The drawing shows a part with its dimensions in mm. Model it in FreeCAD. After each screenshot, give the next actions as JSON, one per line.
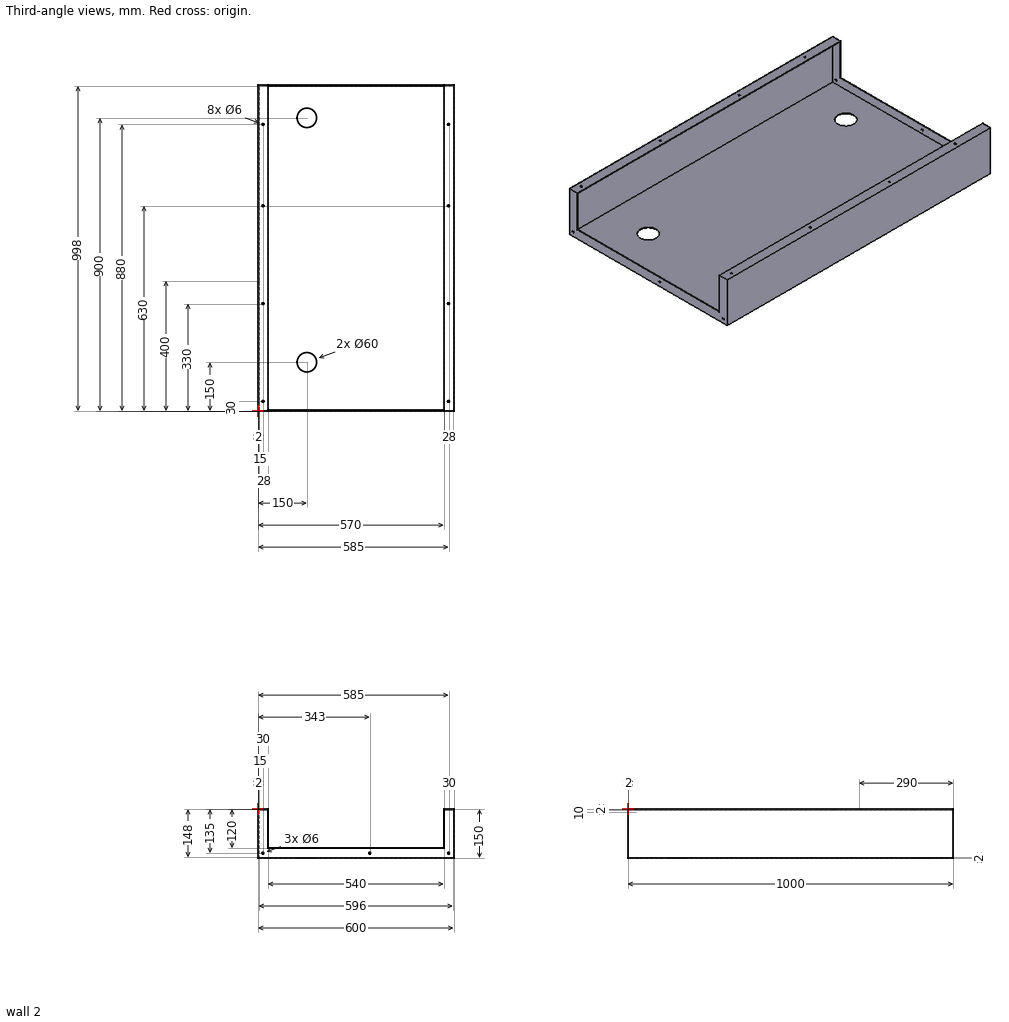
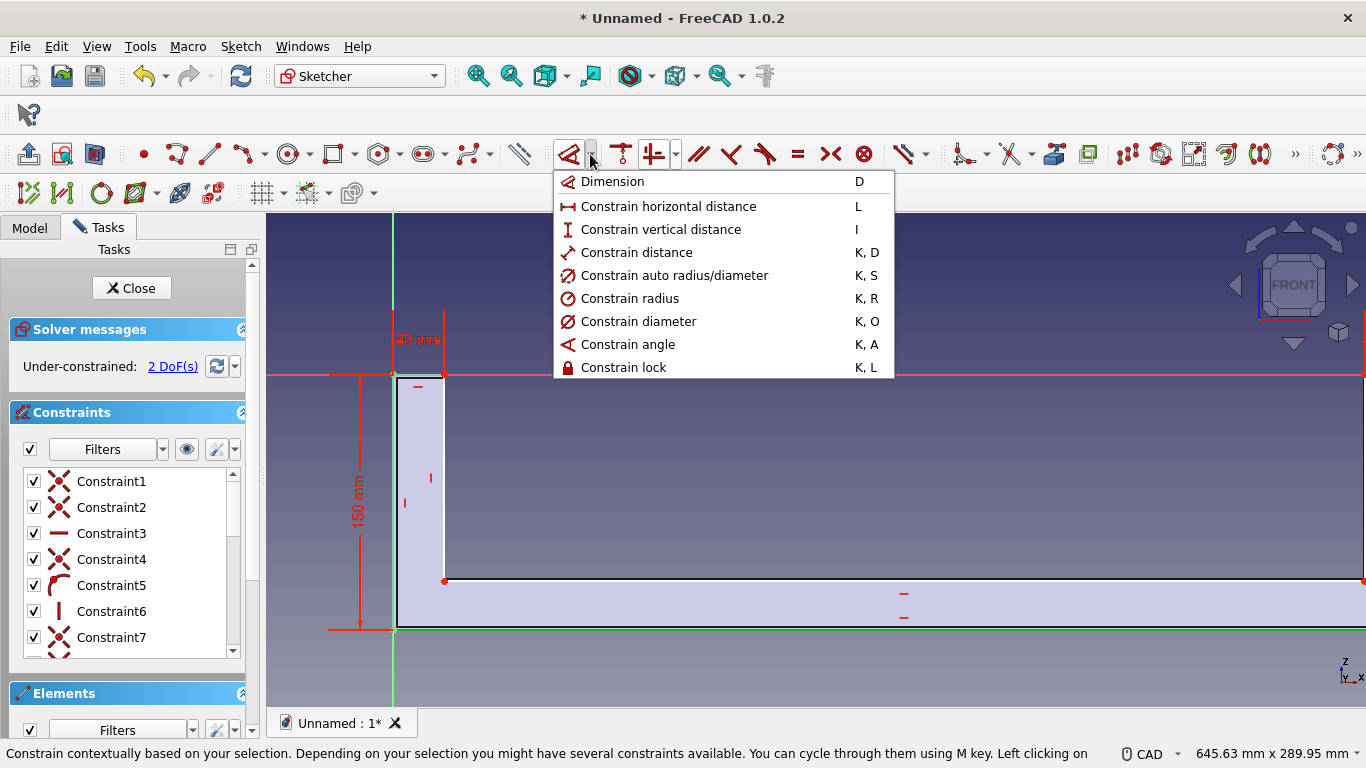
{"action": "left_click", "coordinate": [724, 206]}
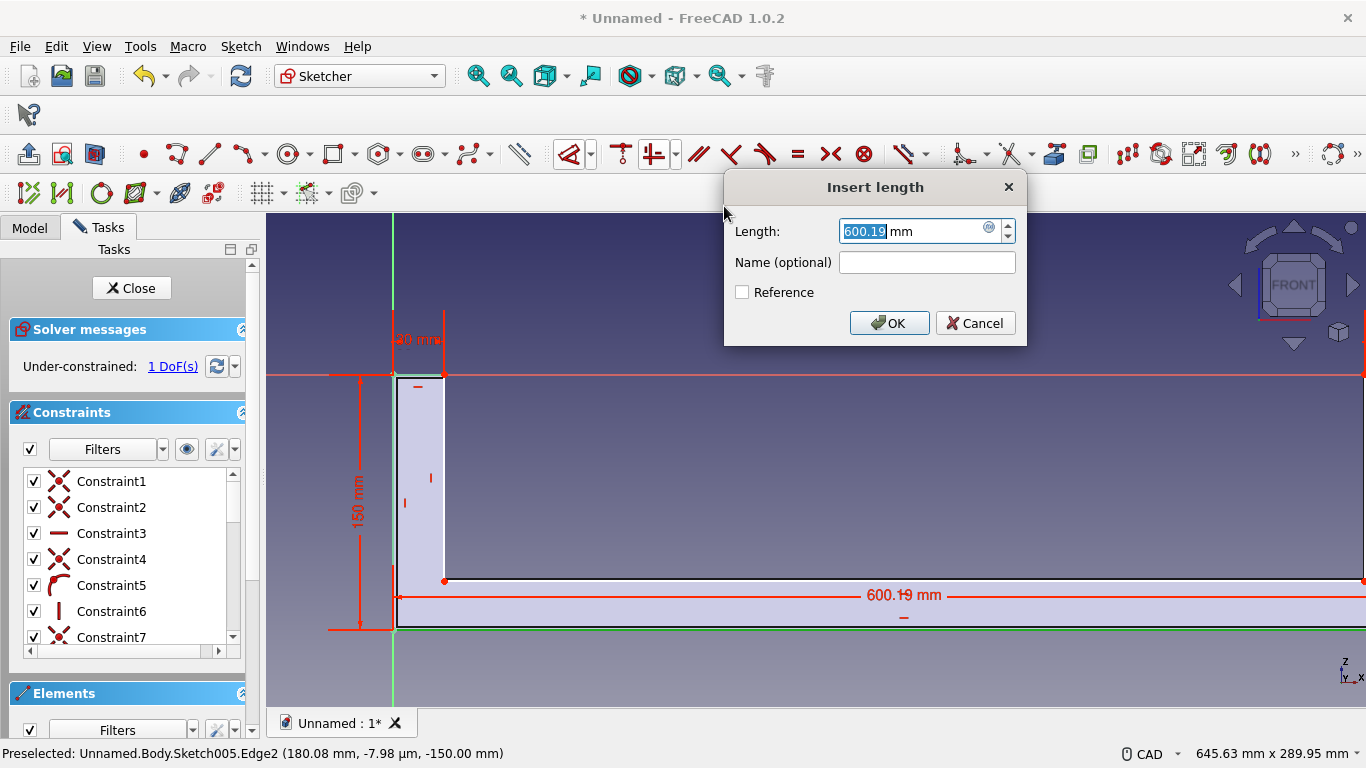
{"action": "type", "text": "600"}
{"action": "key", "text": "Return"}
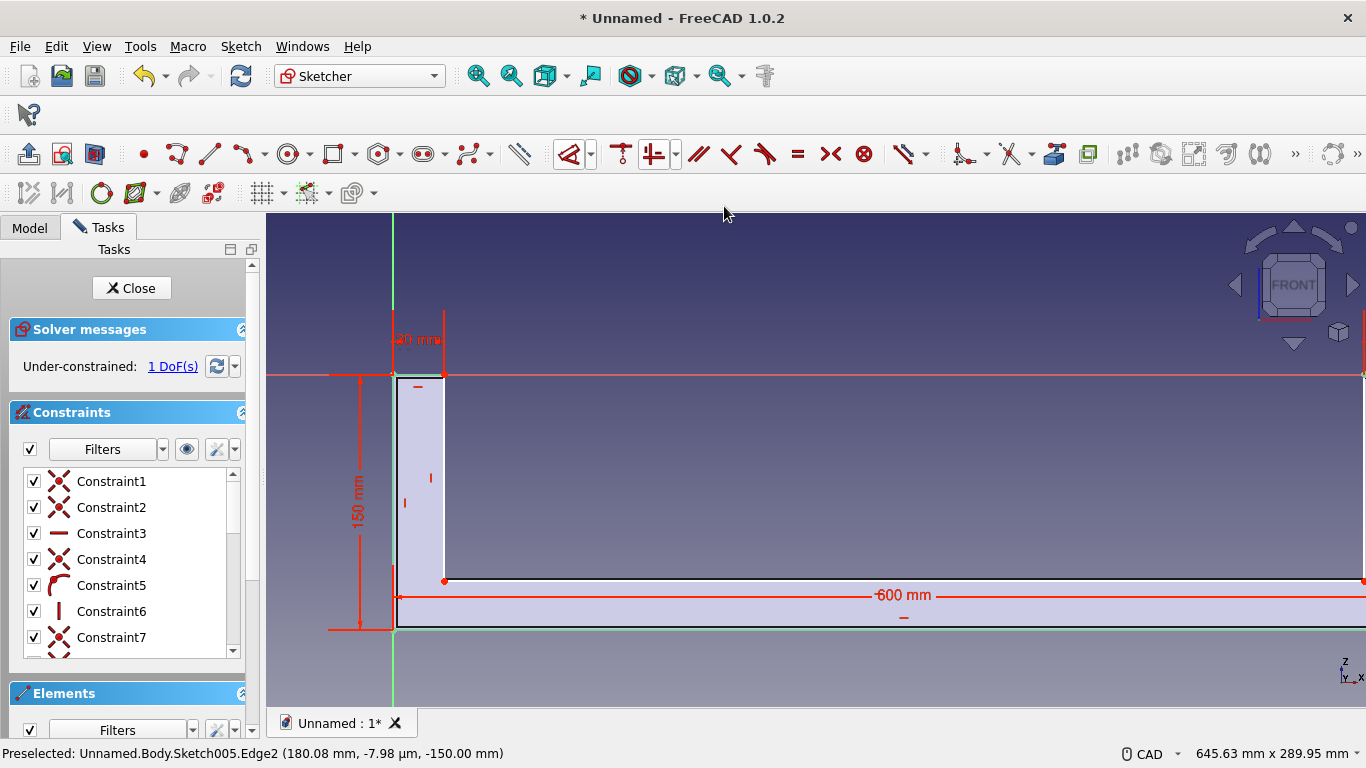
{"action": "scroll", "coordinate": [429, 374], "scroll_direction": "down", "scroll_amount": 2}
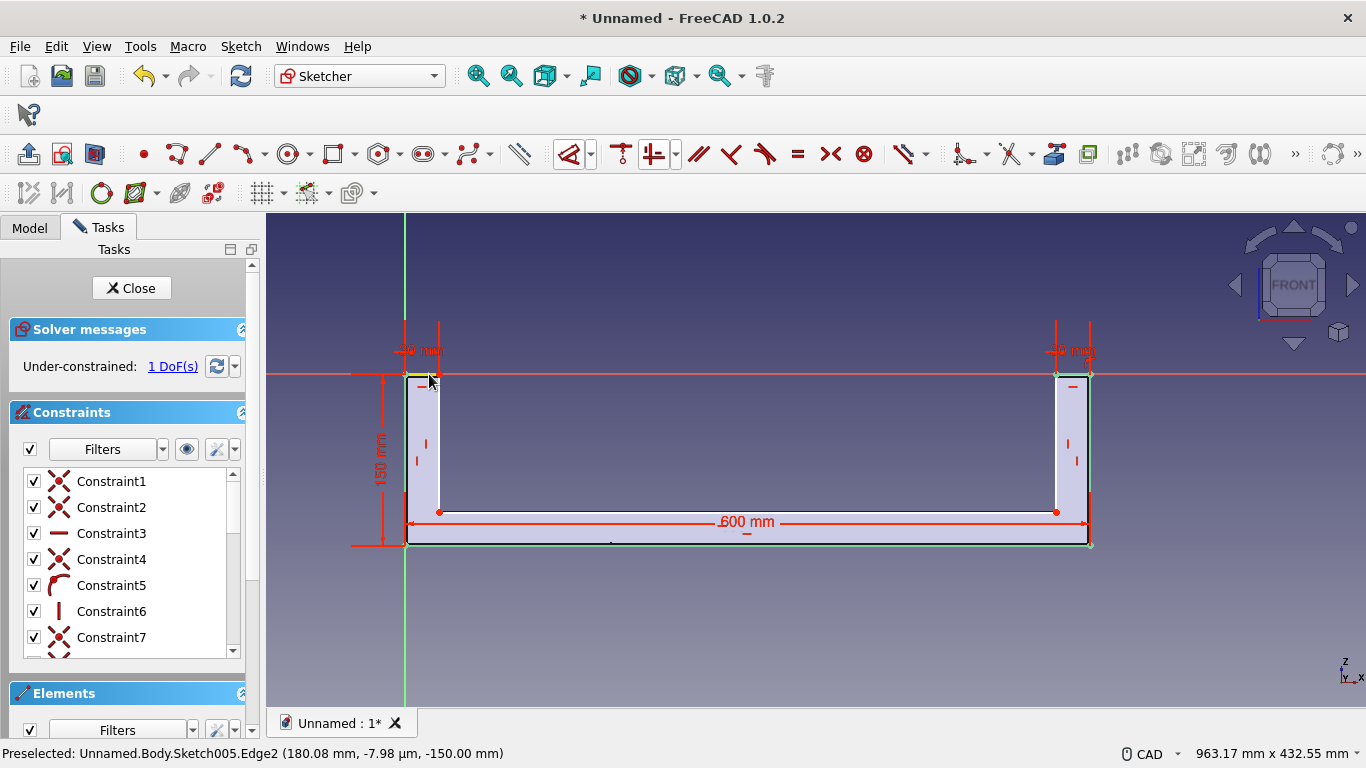
{"action": "left_click", "coordinate": [1056, 416]}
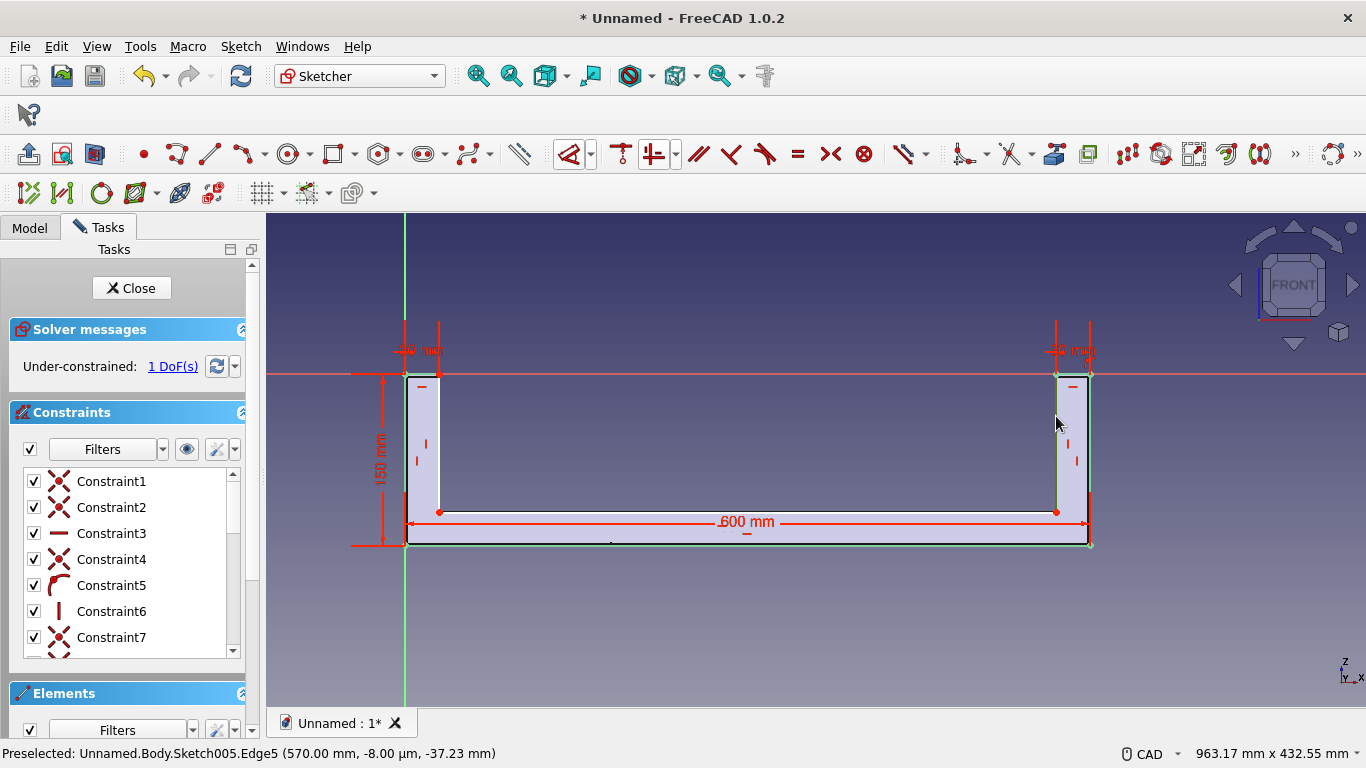
{"action": "left_click", "coordinate": [590, 154]}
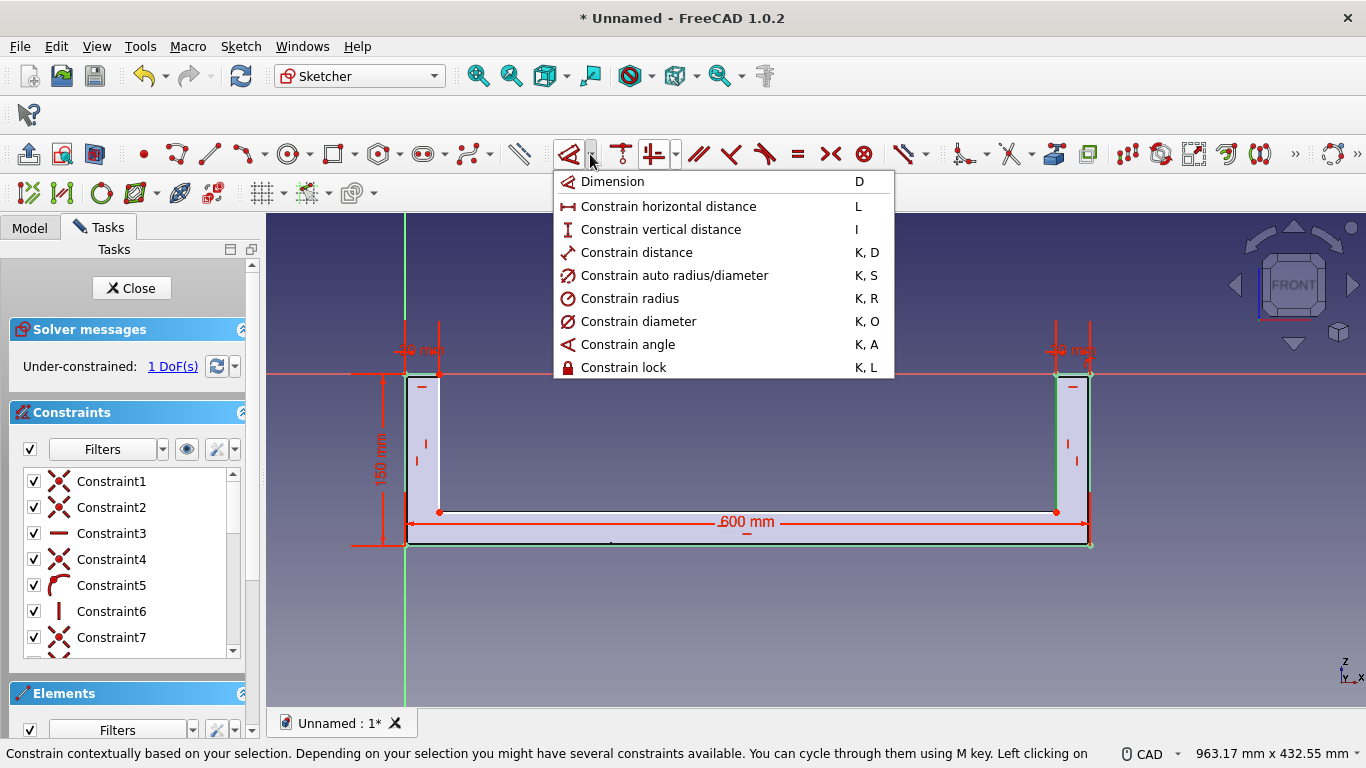
{"action": "left_click", "coordinate": [724, 230]}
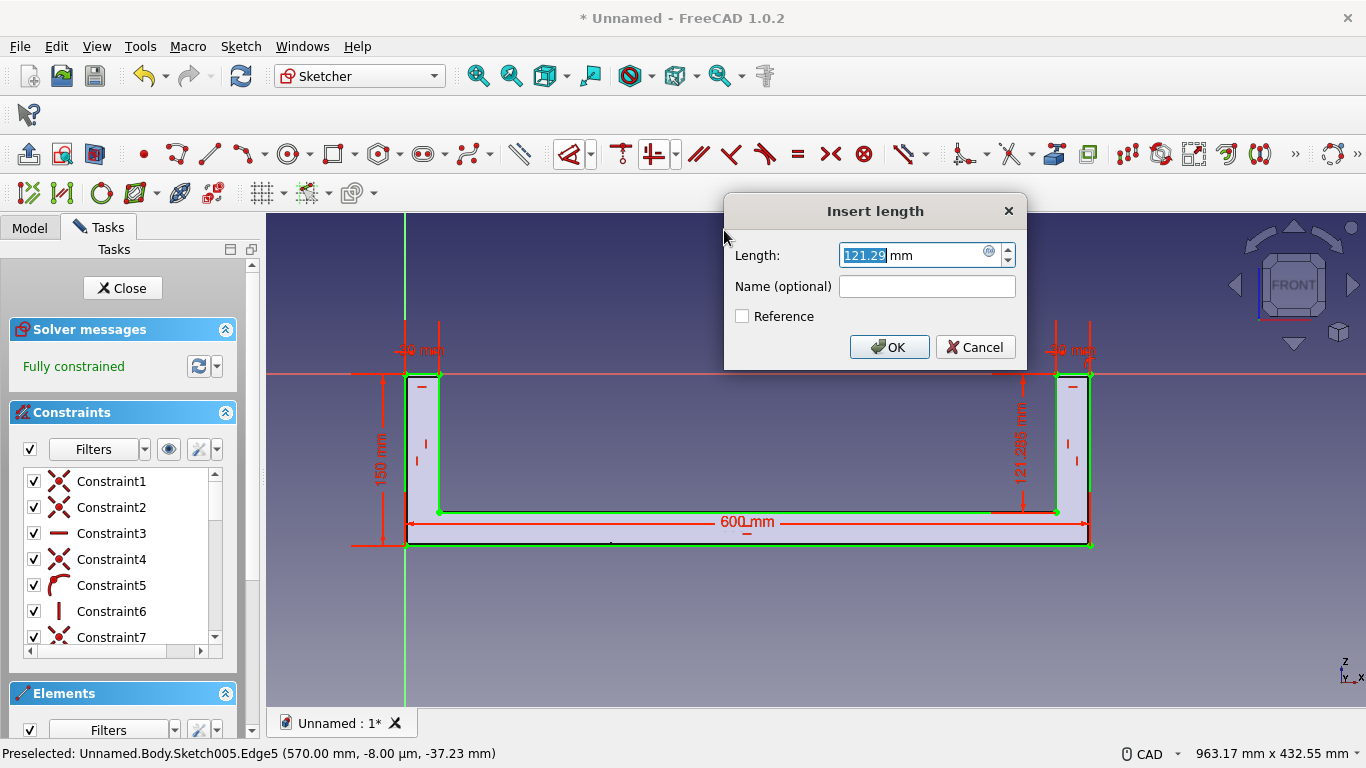
{"action": "type", "text": "120"}
{"action": "key", "text": "Return"}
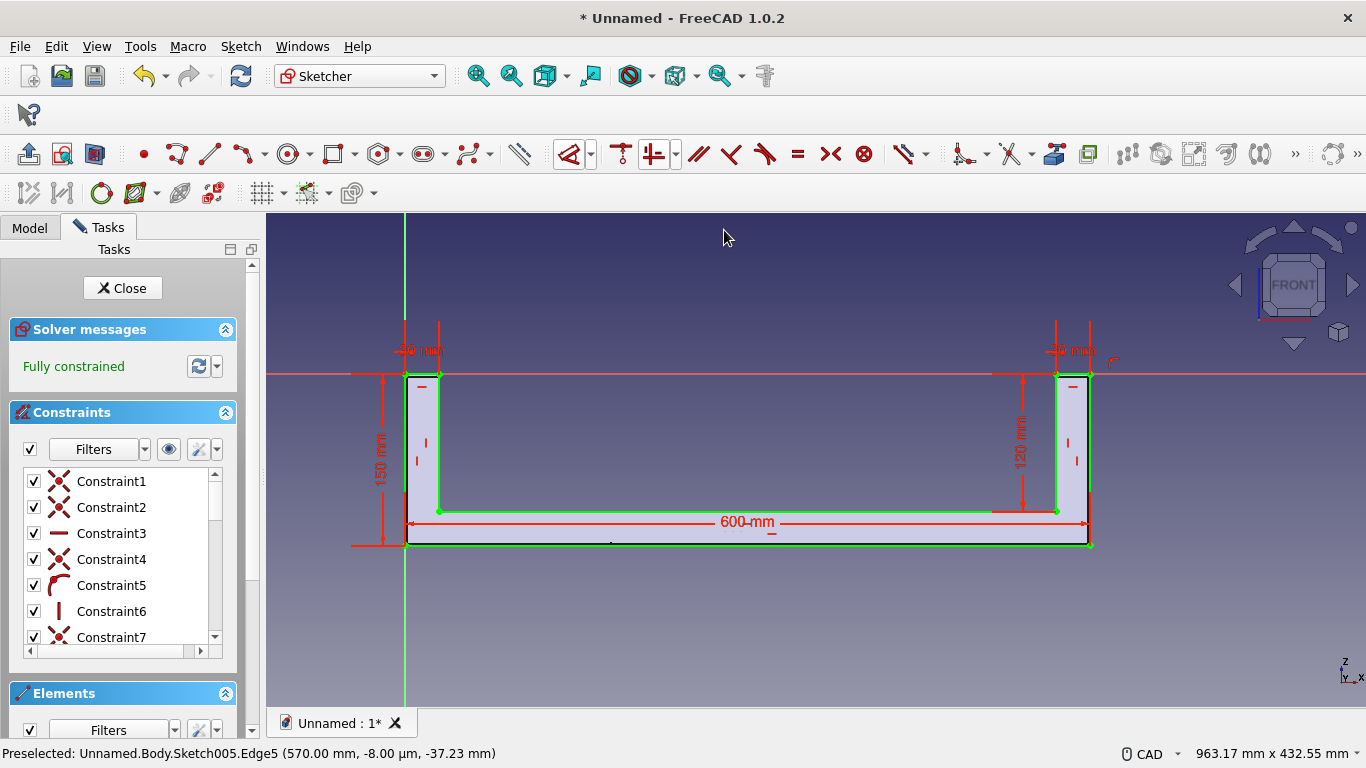
{"action": "left_click", "coordinate": [123, 288]}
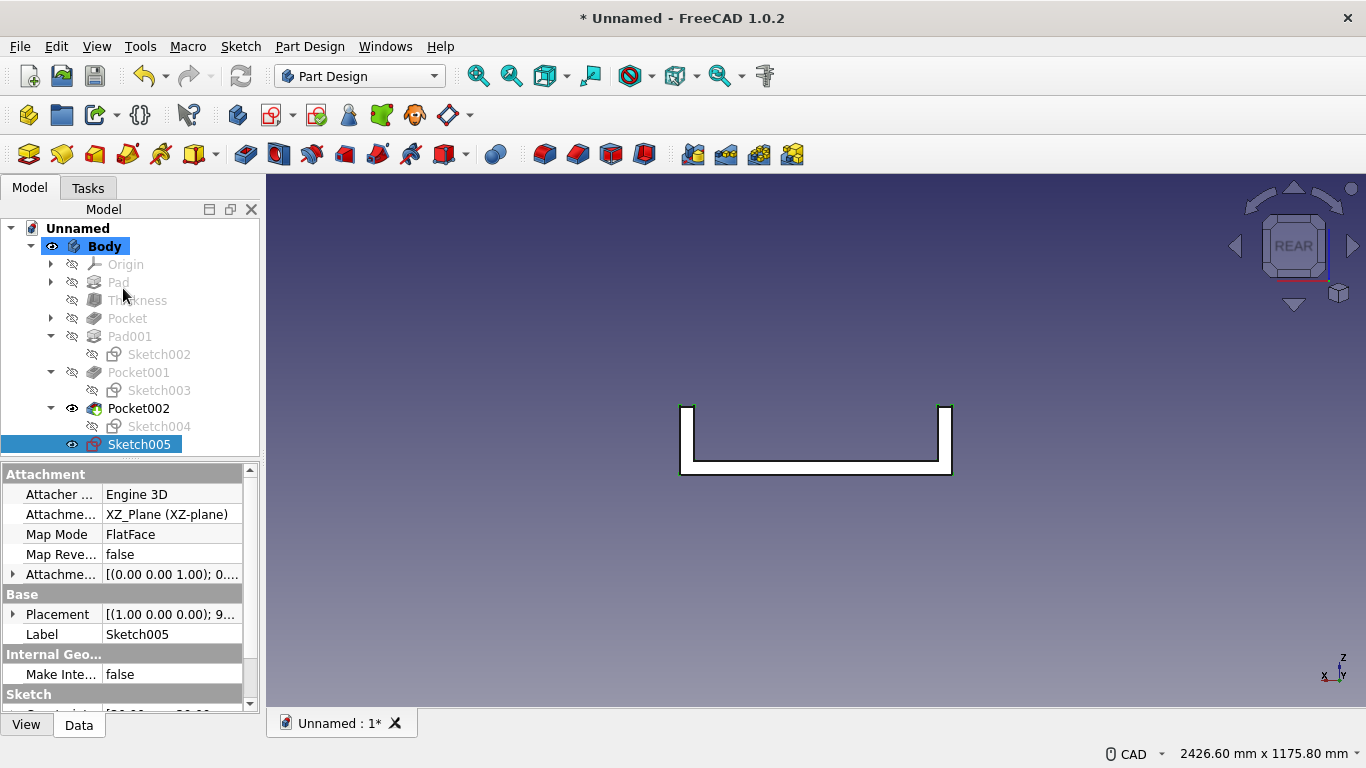
{"action": "left_click", "coordinate": [29, 154]}